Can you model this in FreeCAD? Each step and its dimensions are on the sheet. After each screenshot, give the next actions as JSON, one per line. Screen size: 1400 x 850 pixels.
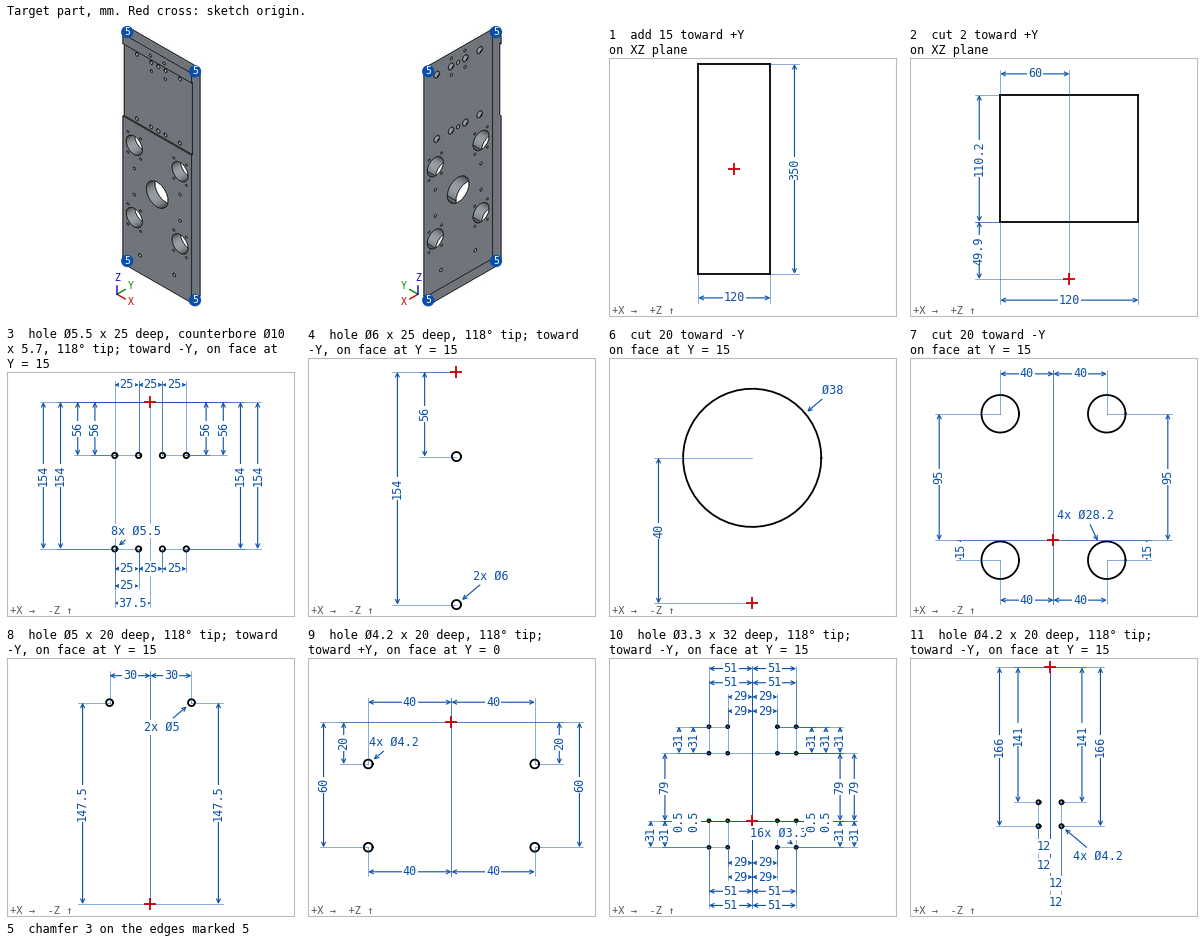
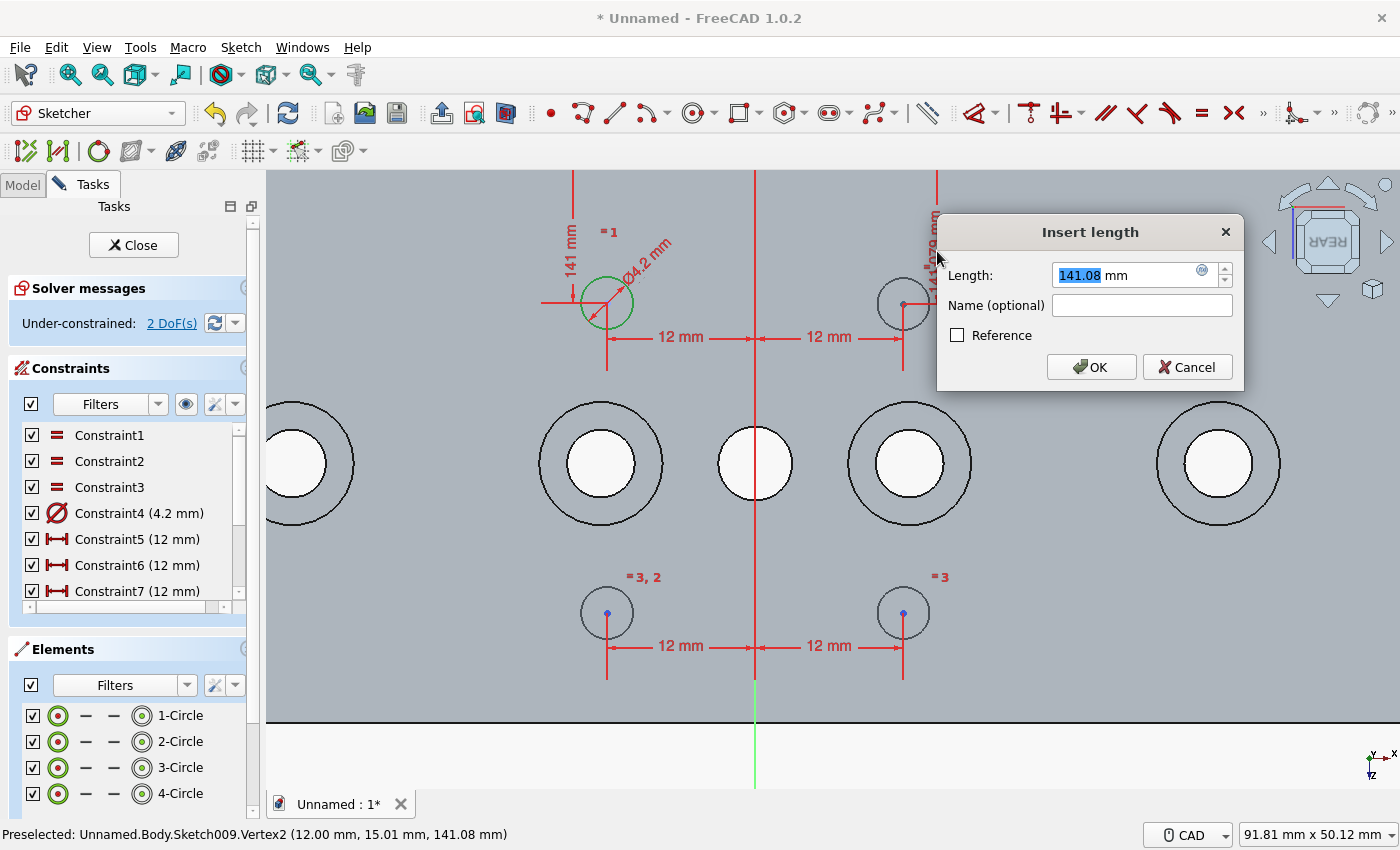
{"action": "type", "text": "141"}
{"action": "key", "text": "Return"}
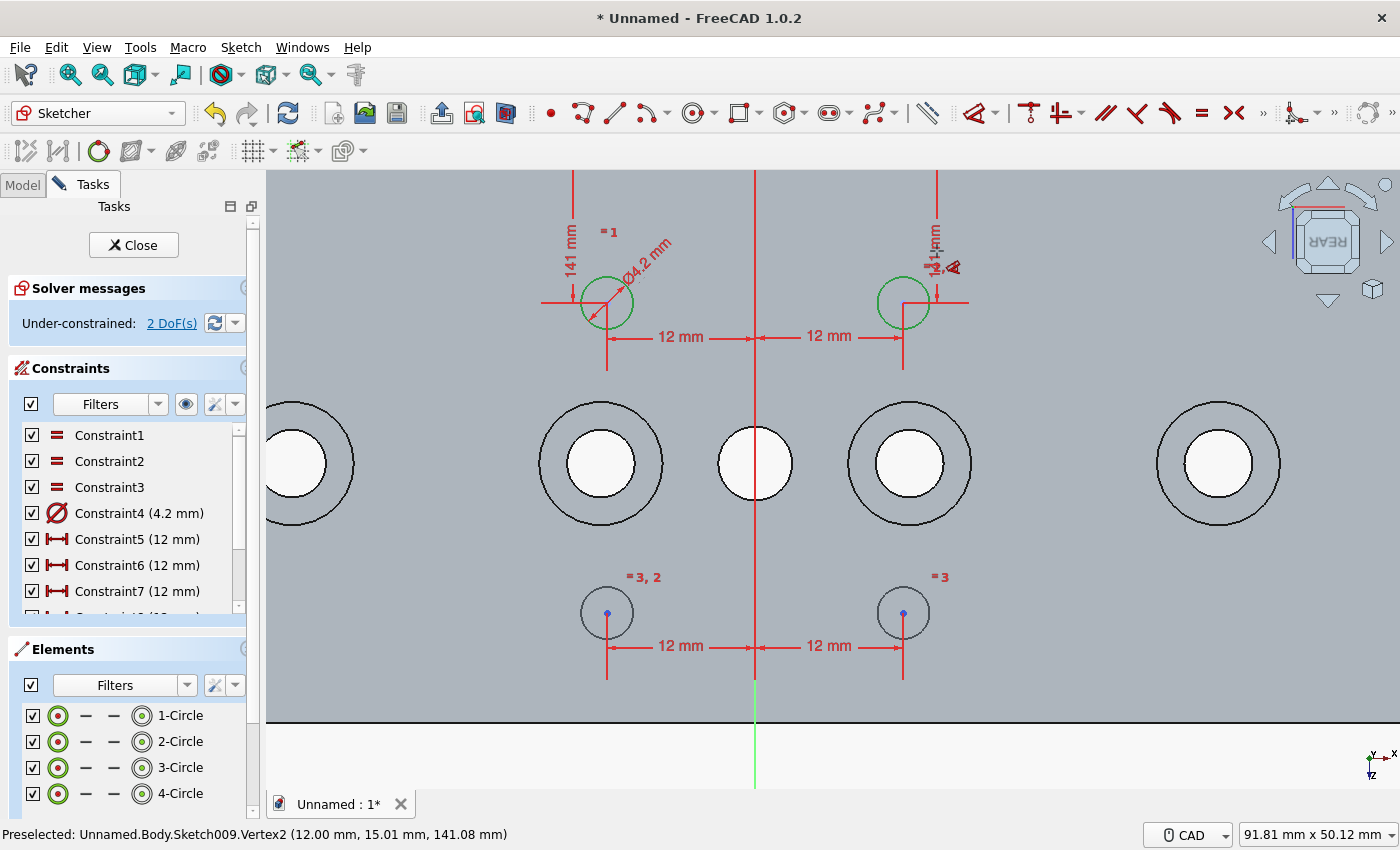
{"action": "left_click", "coordinate": [607, 613]}
{"action": "left_click", "coordinate": [573, 405]}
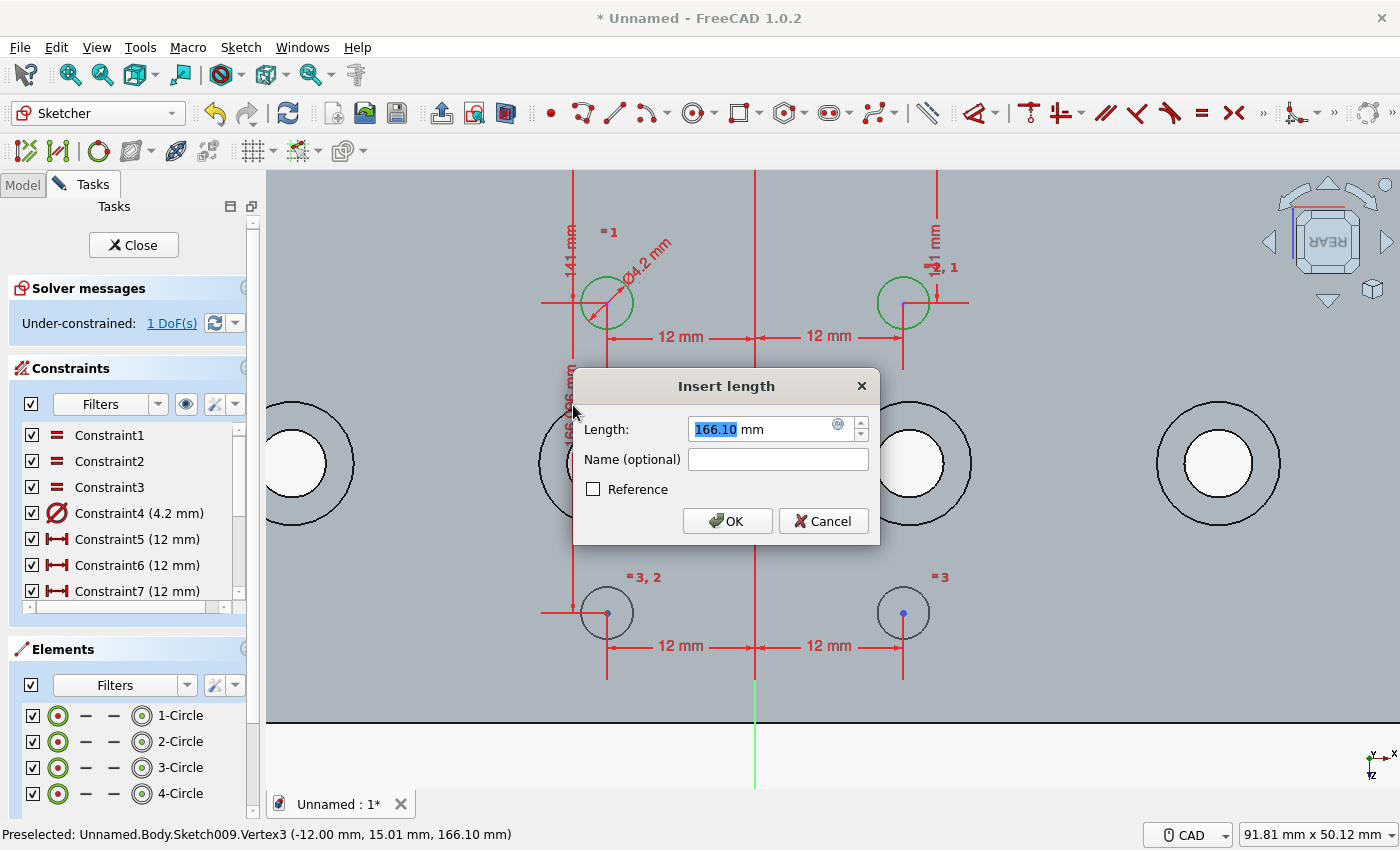
{"action": "type", "text": "166"}
{"action": "key", "text": "Return"}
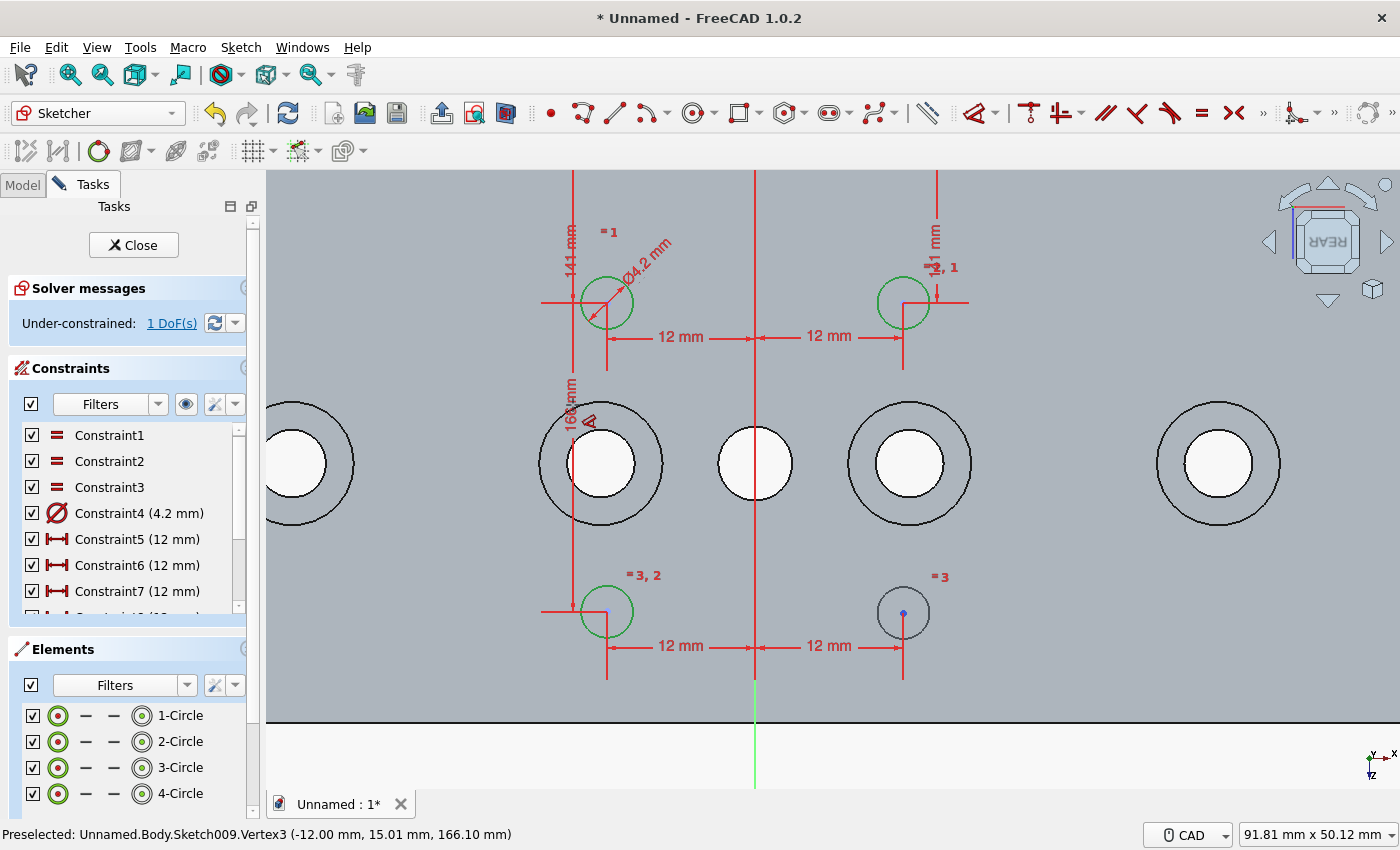
{"action": "left_click", "coordinate": [903, 613]}
{"action": "left_click", "coordinate": [937, 405]}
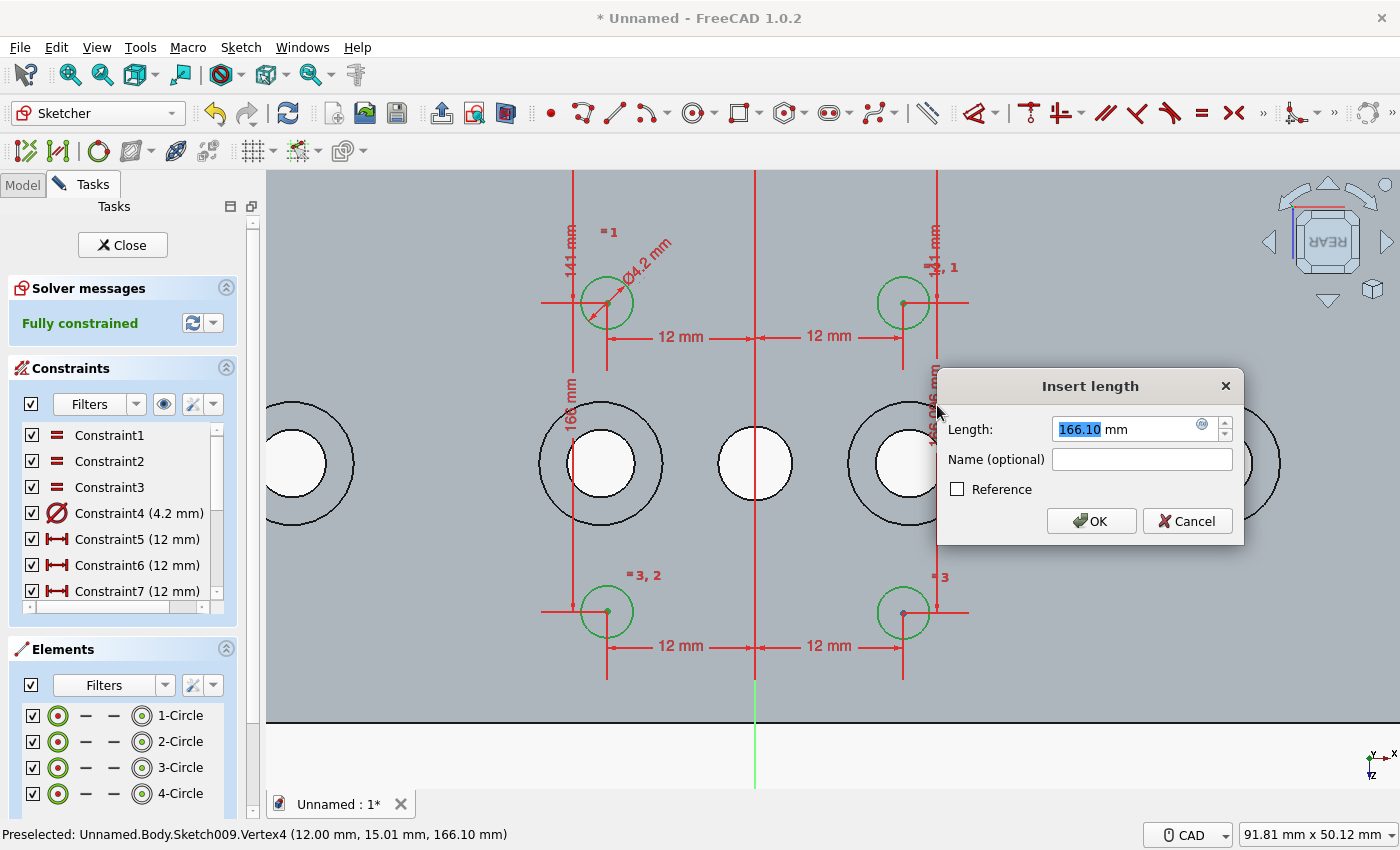
{"action": "type", "text": "166"}
{"action": "key", "text": "Return"}
{"action": "key", "text": "Escape"}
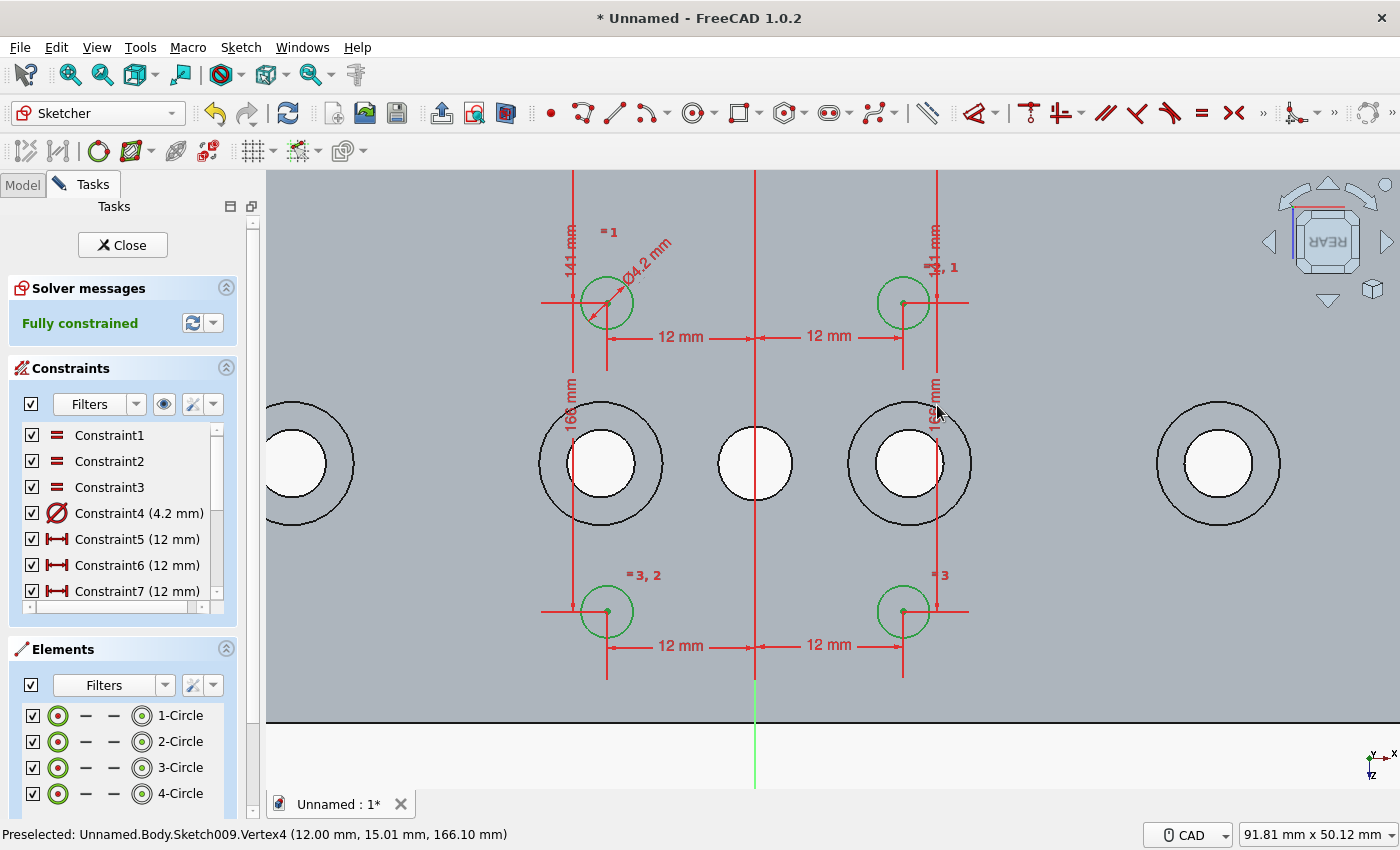
{"action": "left_click", "coordinate": [123, 245]}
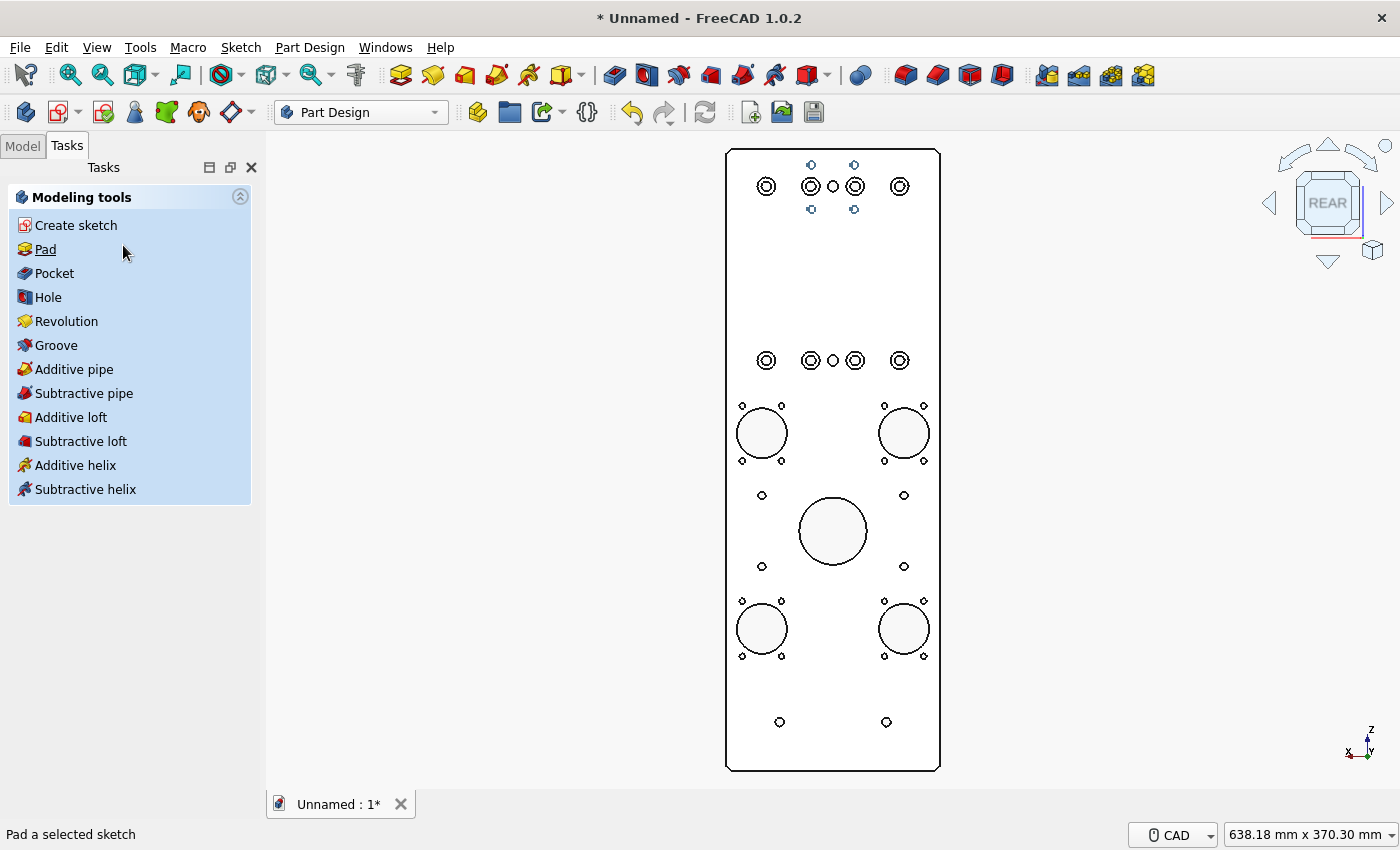
{"action": "left_click", "coordinate": [648, 76]}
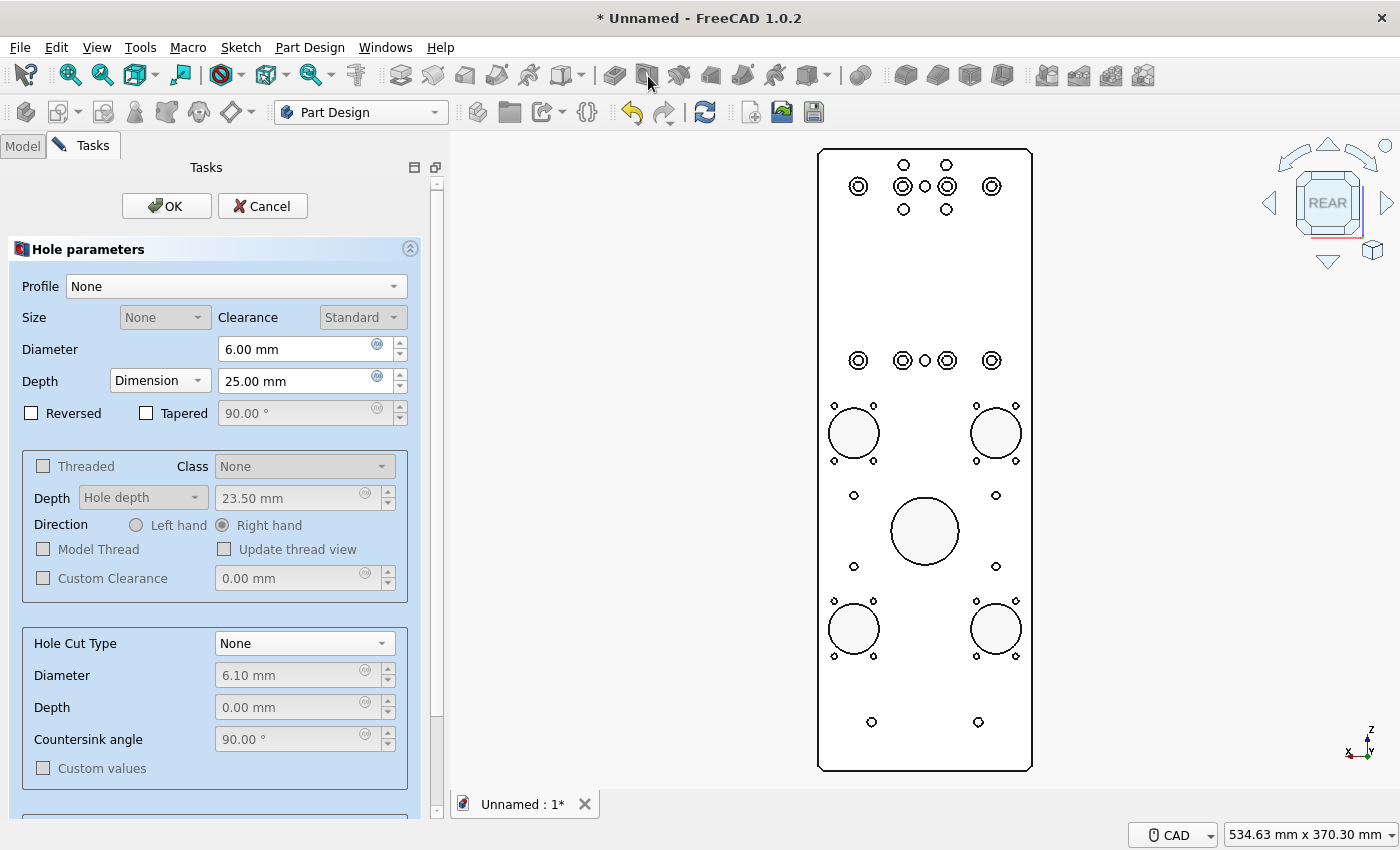
{"action": "triple_click", "coordinate": [305, 349]}